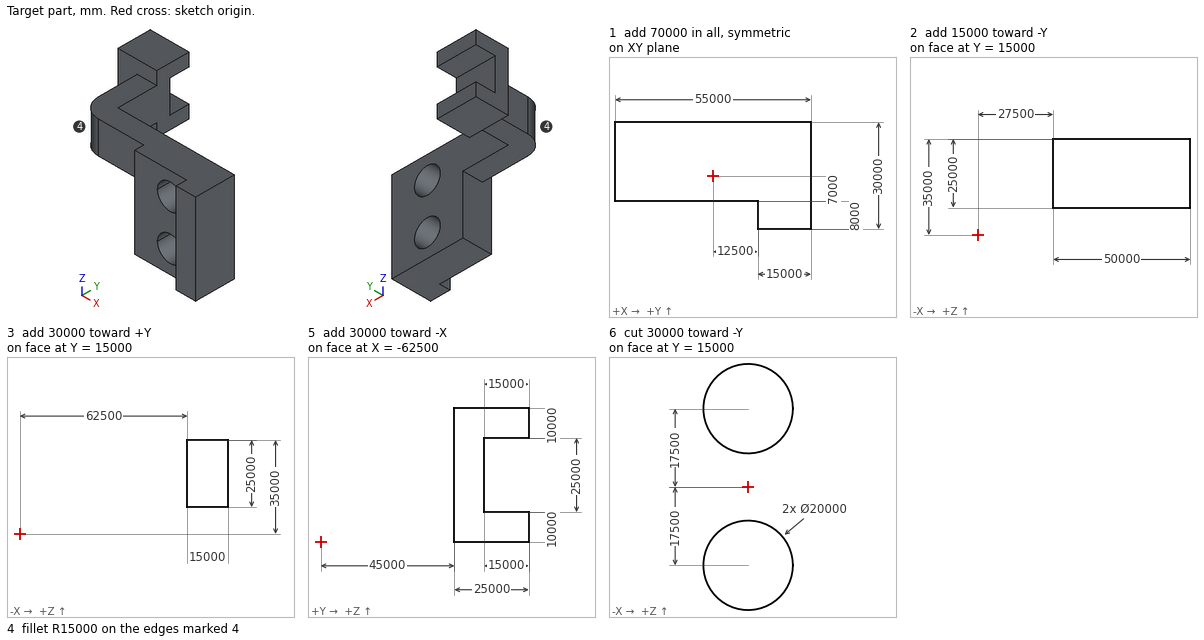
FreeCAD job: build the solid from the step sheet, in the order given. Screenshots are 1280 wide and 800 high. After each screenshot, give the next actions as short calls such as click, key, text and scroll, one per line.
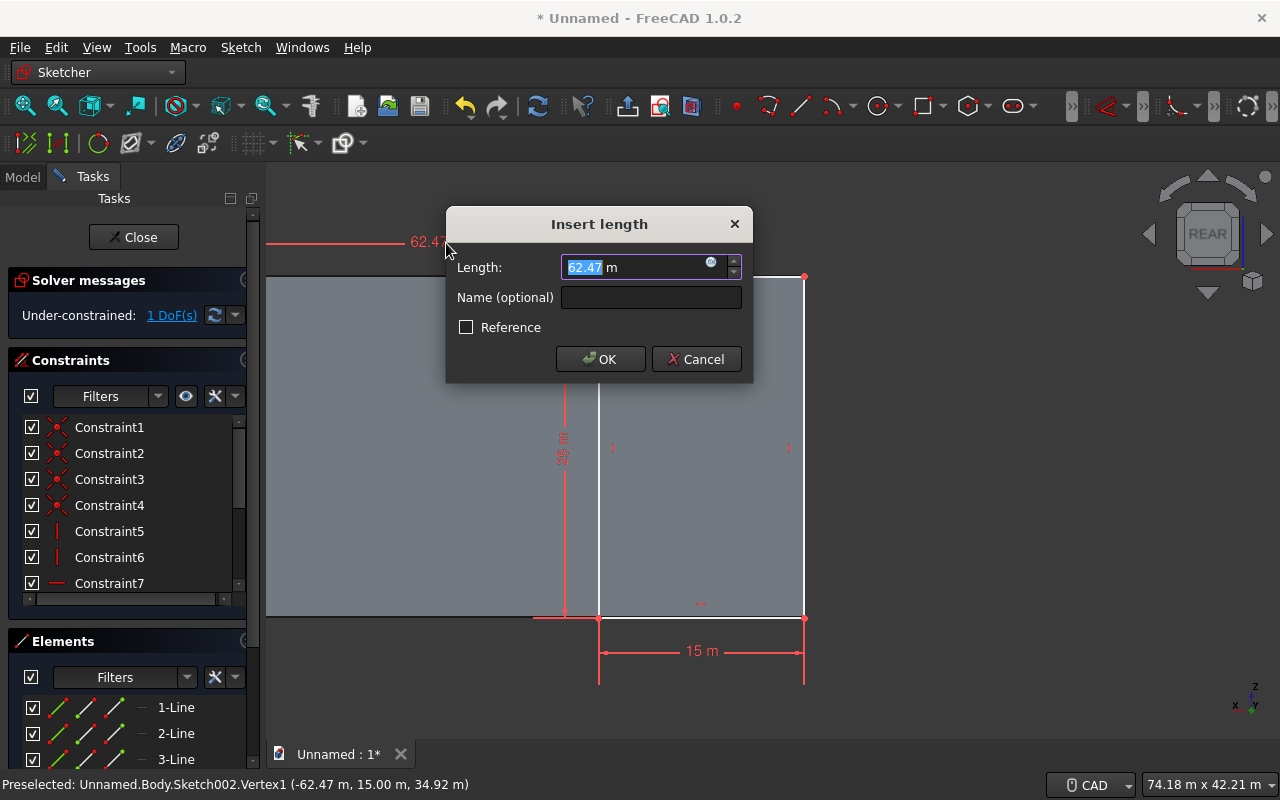
key(ctrl+a)
text(62500 mm)
key(Return)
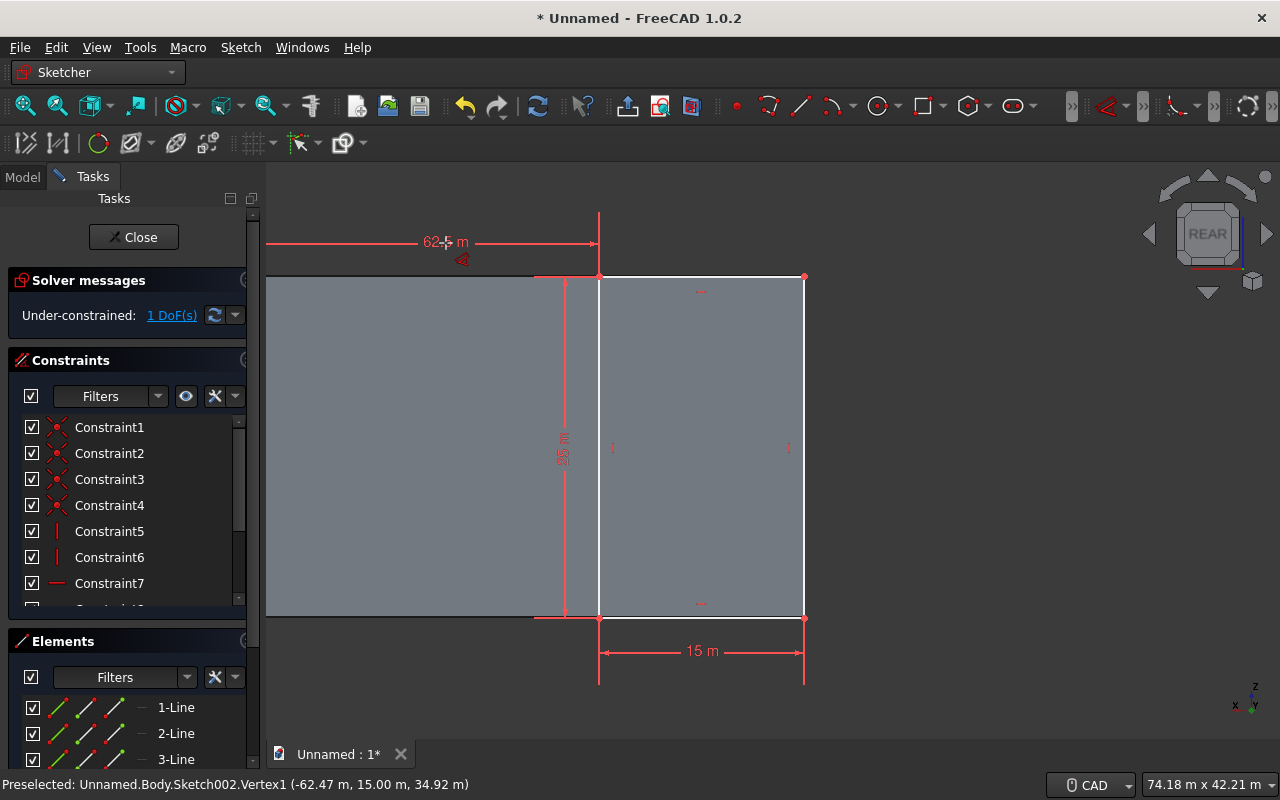
click(599, 277)
click(633, 494)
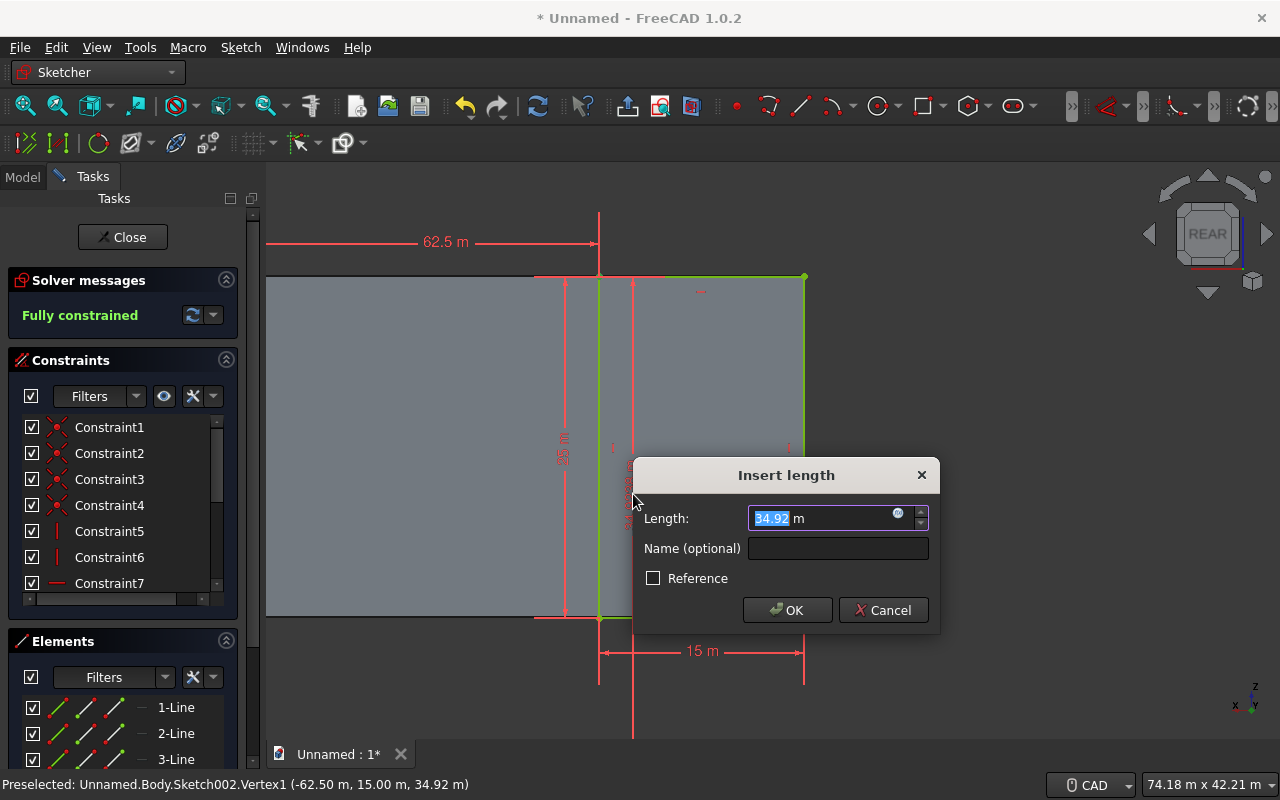
key(ctrl+a)
text(35000 mm)
key(Return)
key(Escape)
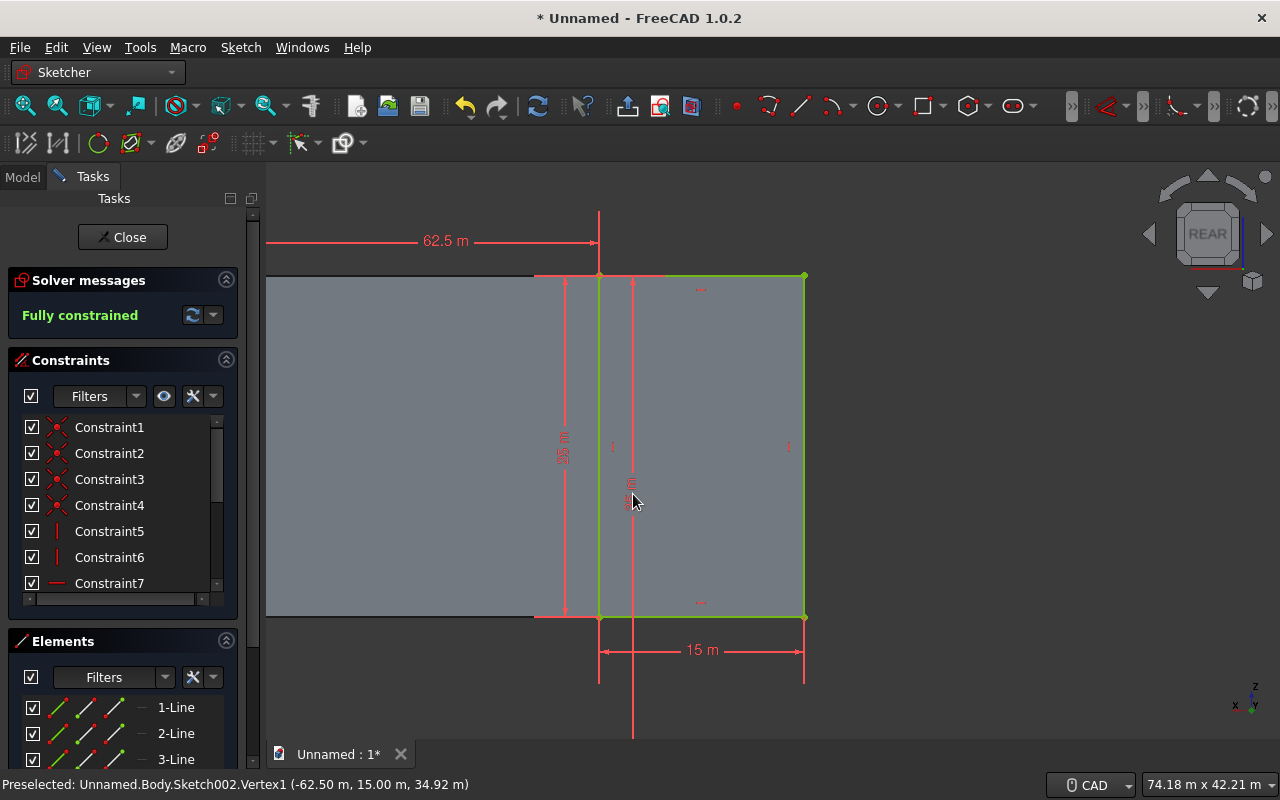
click(123, 237)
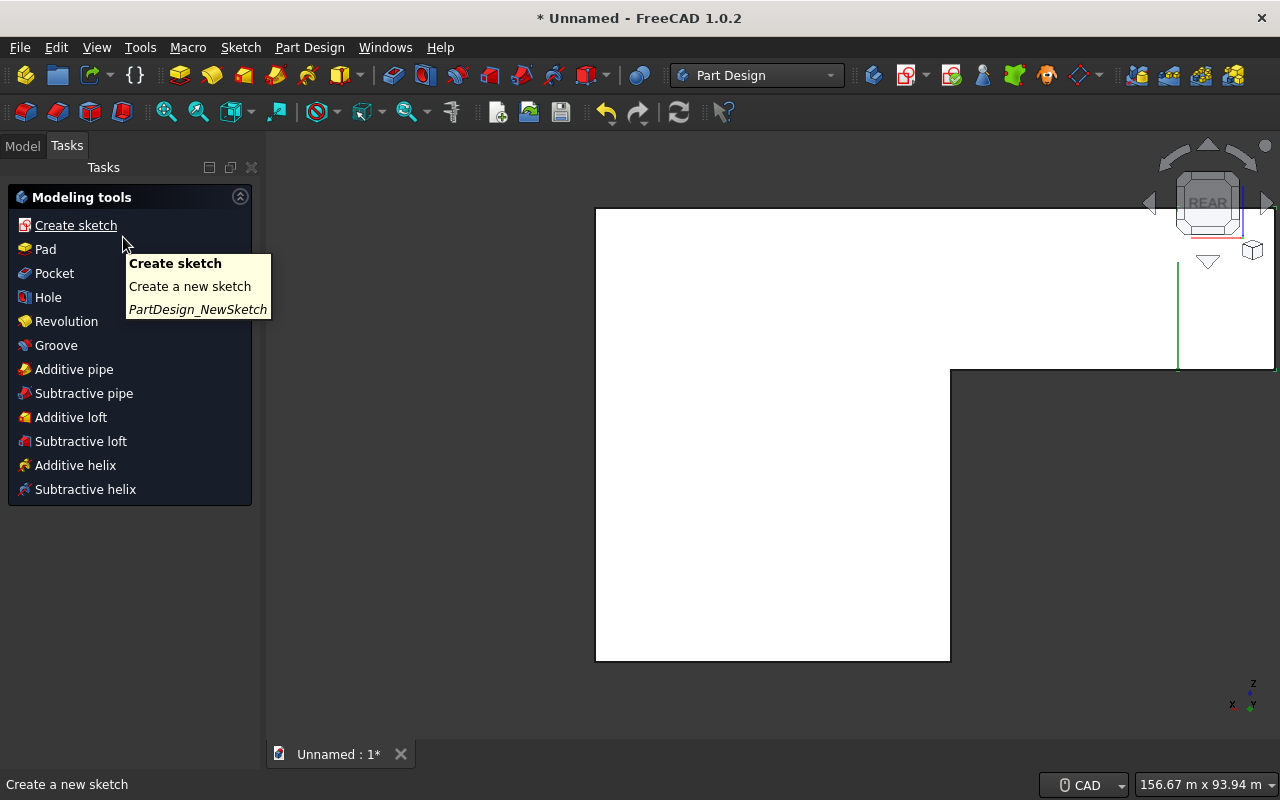
click(180, 76)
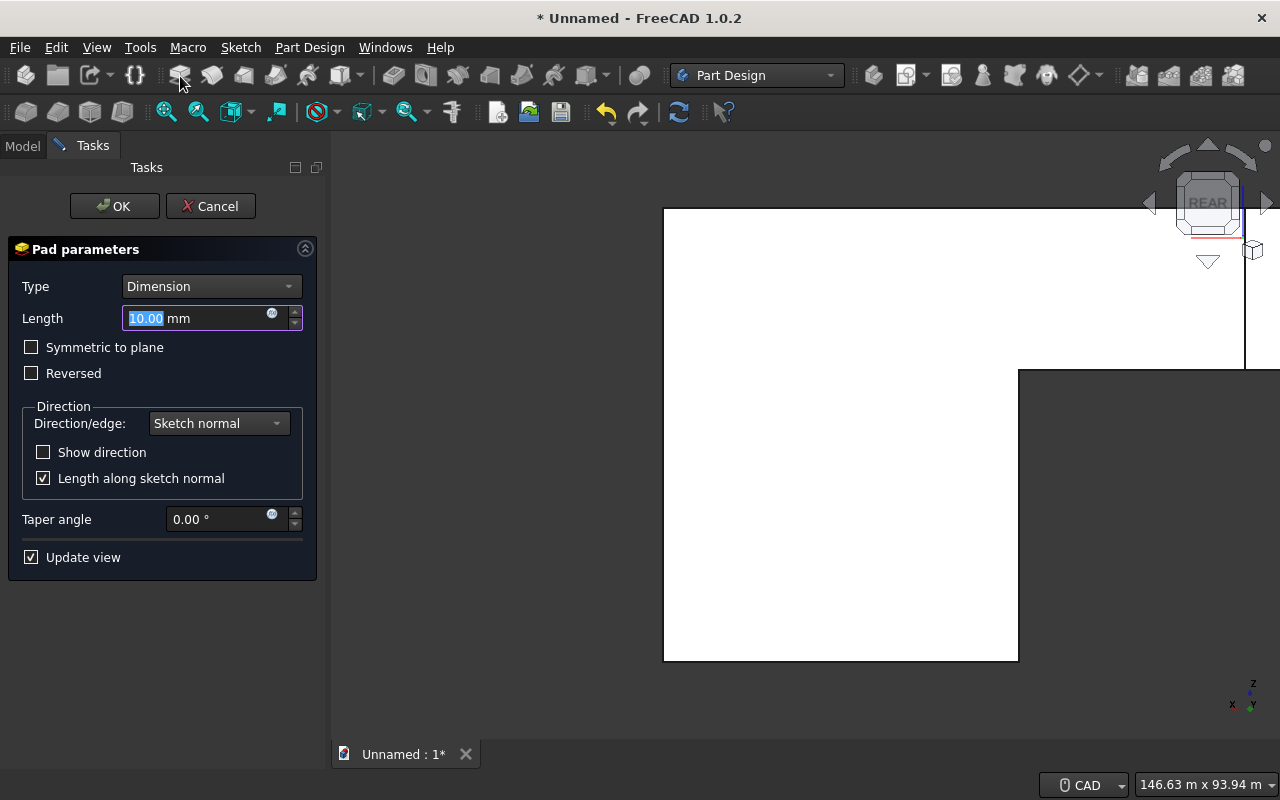
text(30000)
key(Tab)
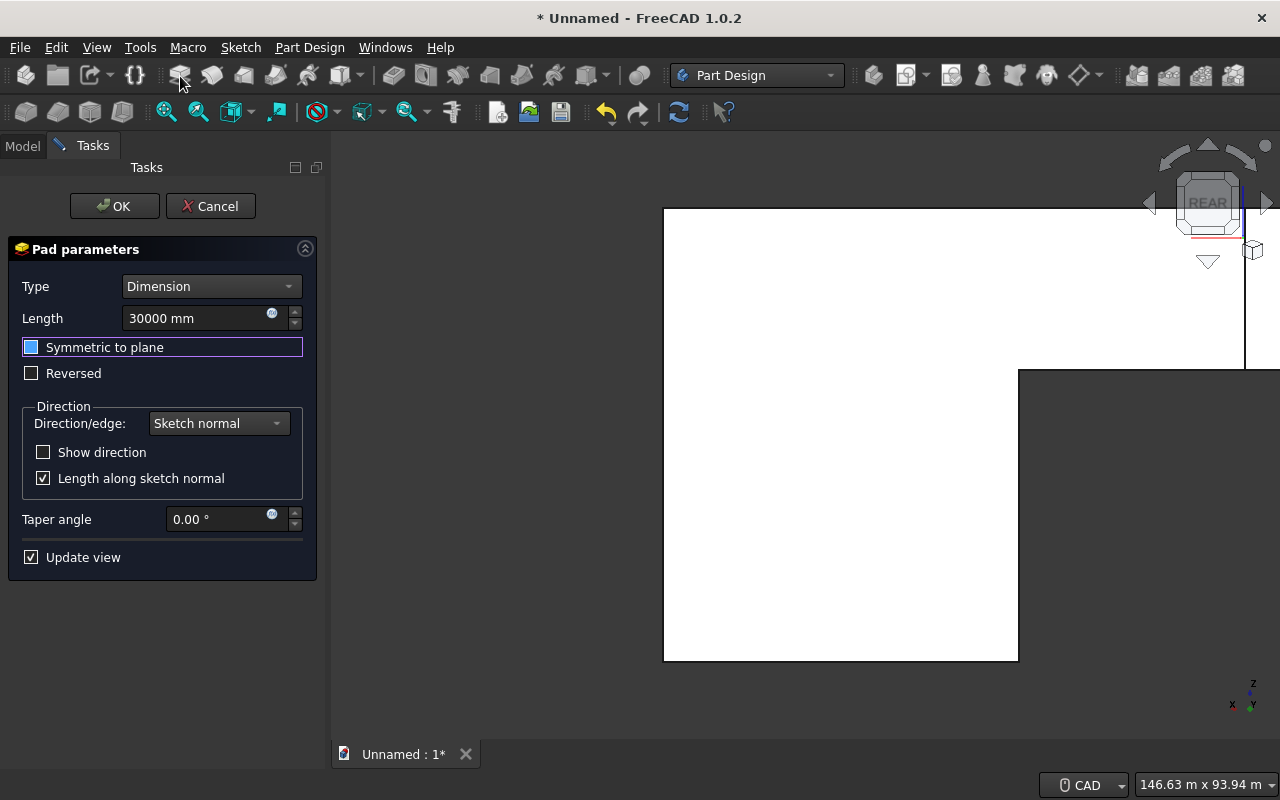
click(115, 206)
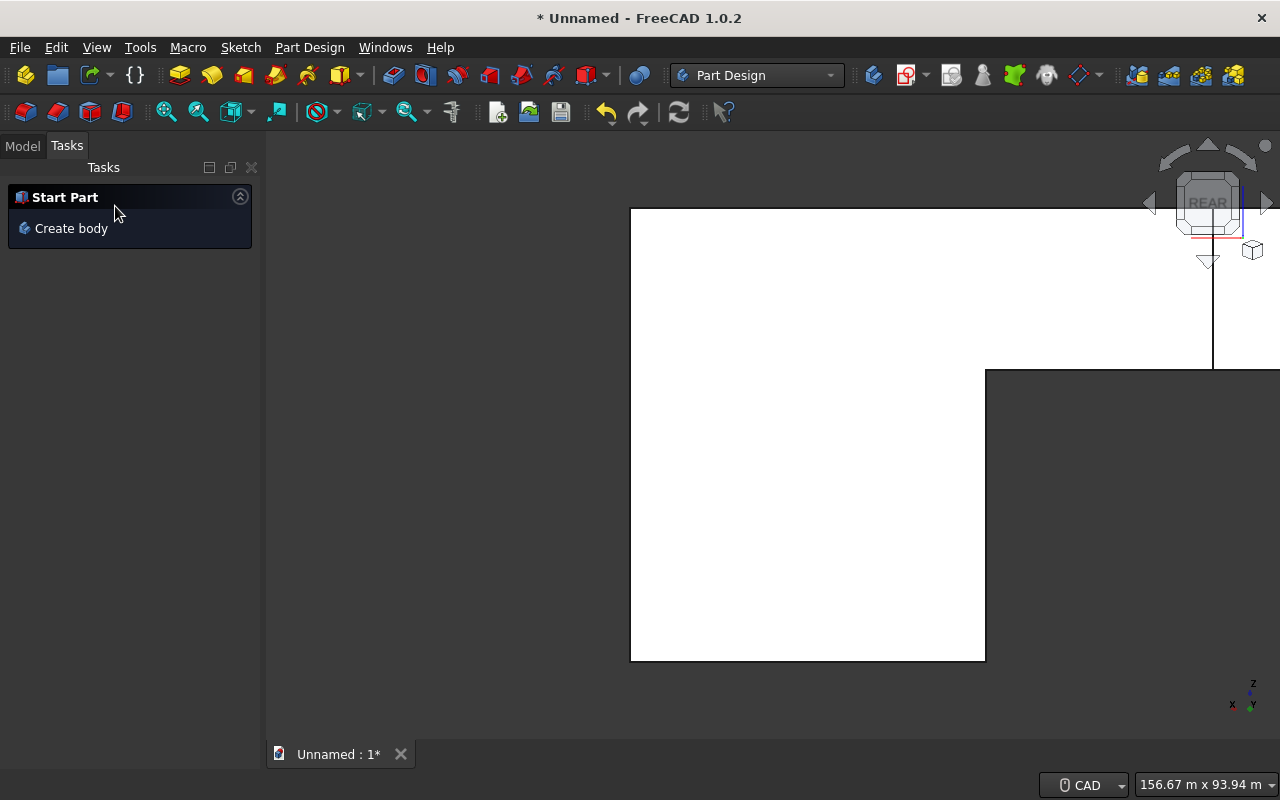
key(v)
key(f)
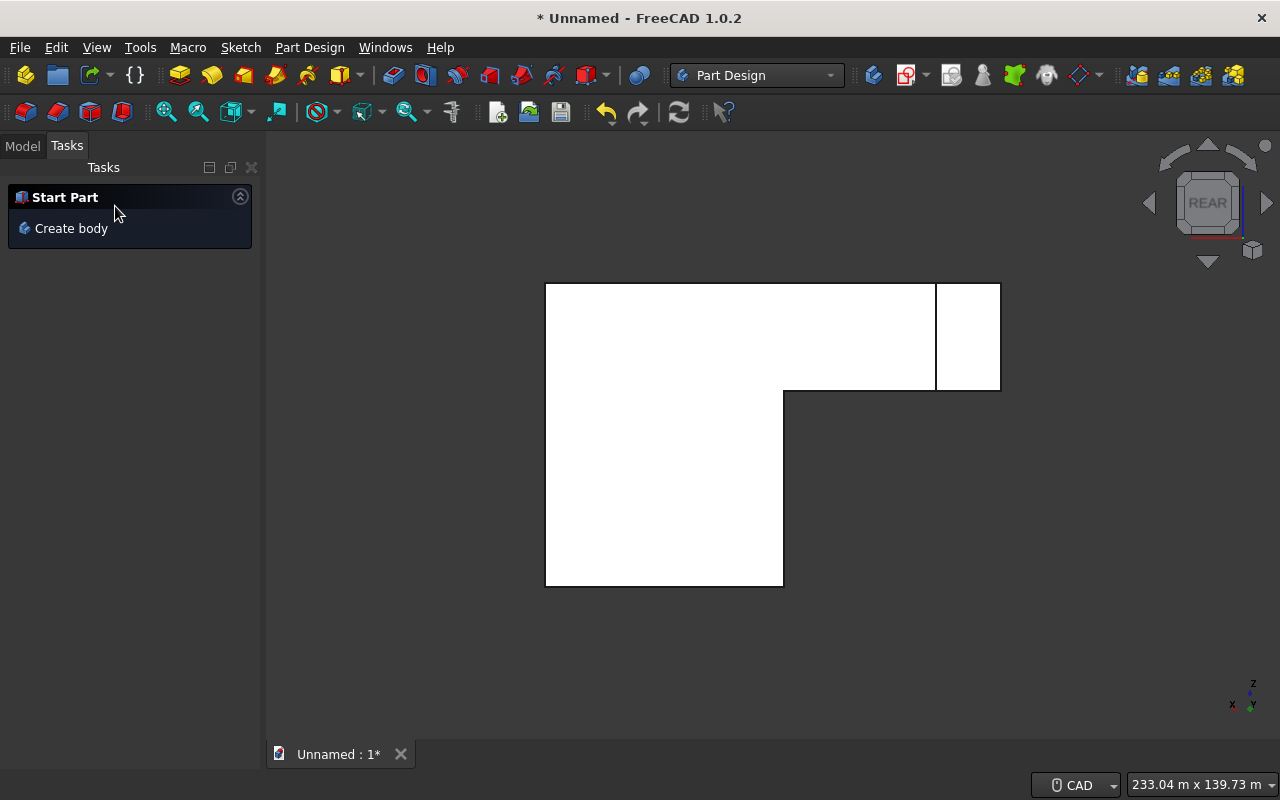
key(0)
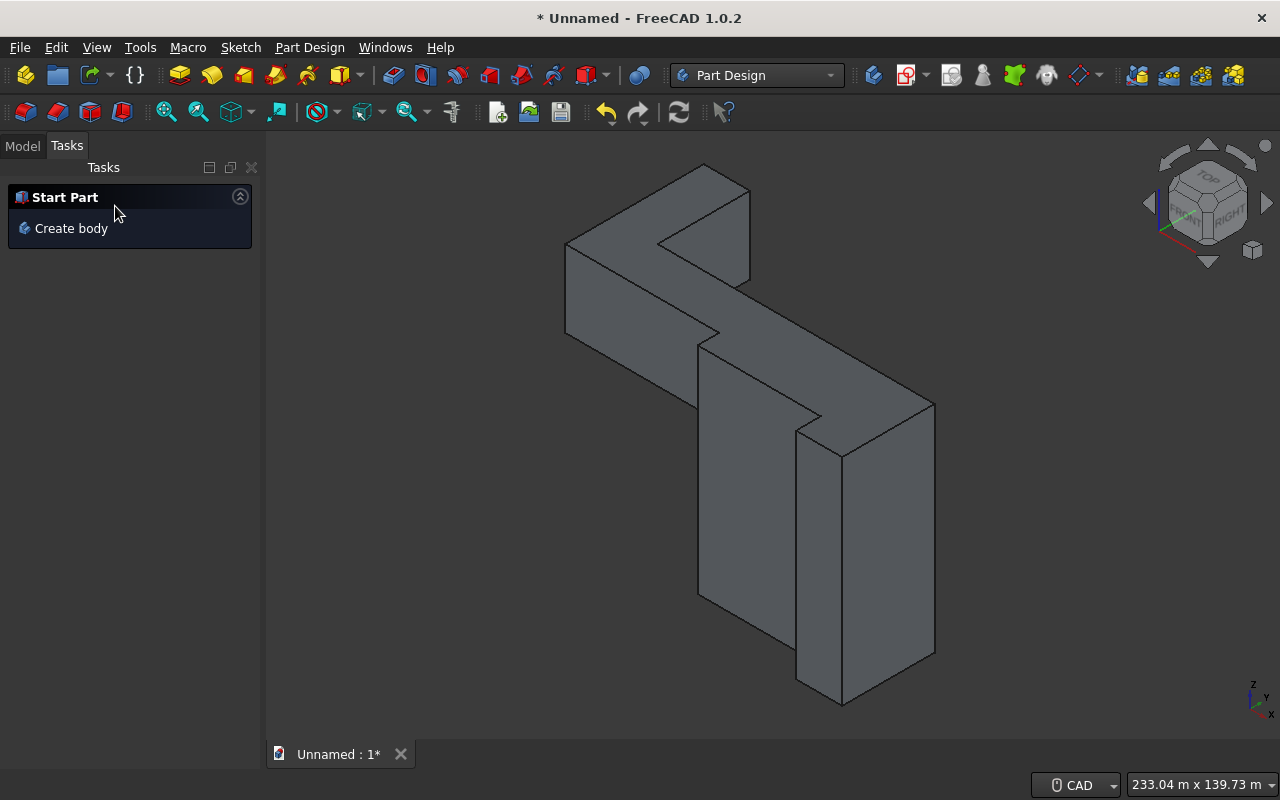
key(2)